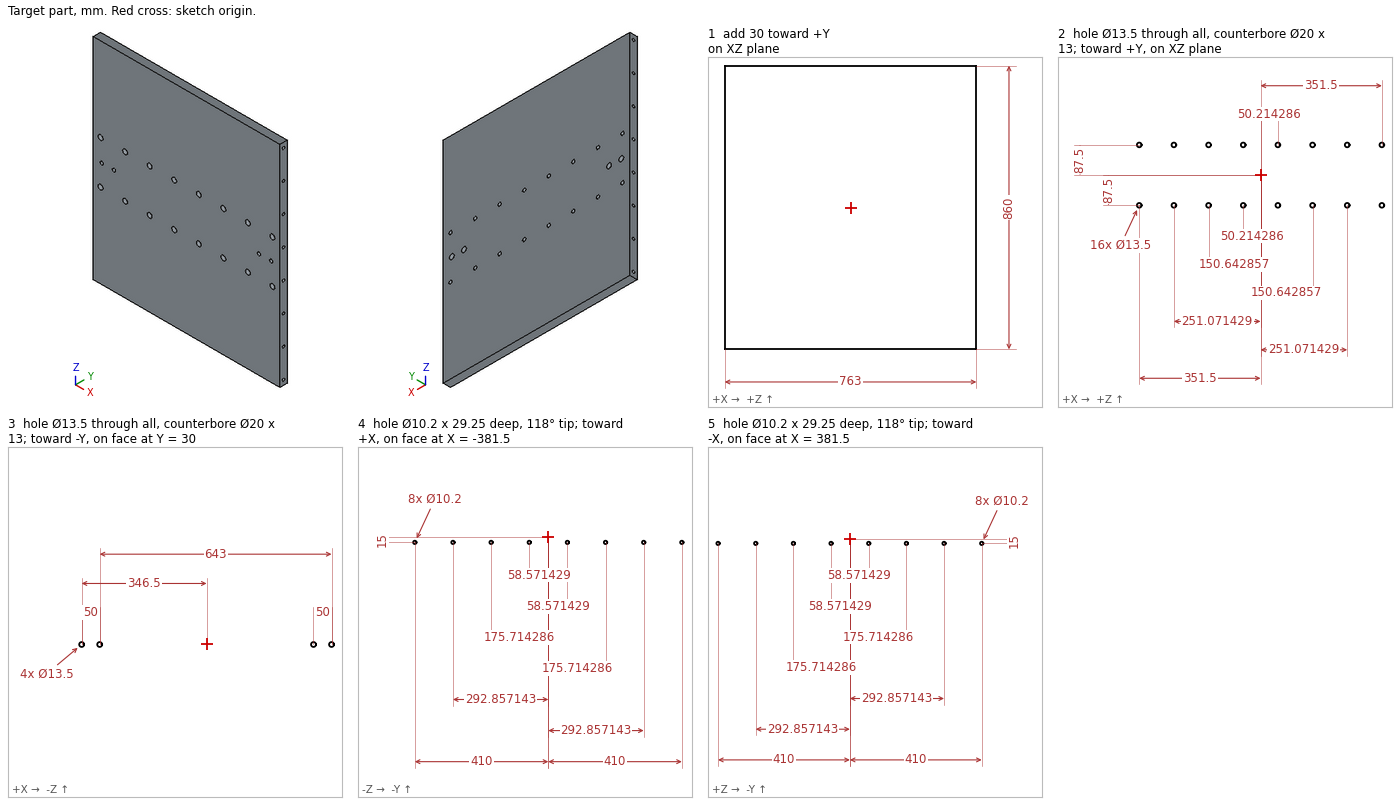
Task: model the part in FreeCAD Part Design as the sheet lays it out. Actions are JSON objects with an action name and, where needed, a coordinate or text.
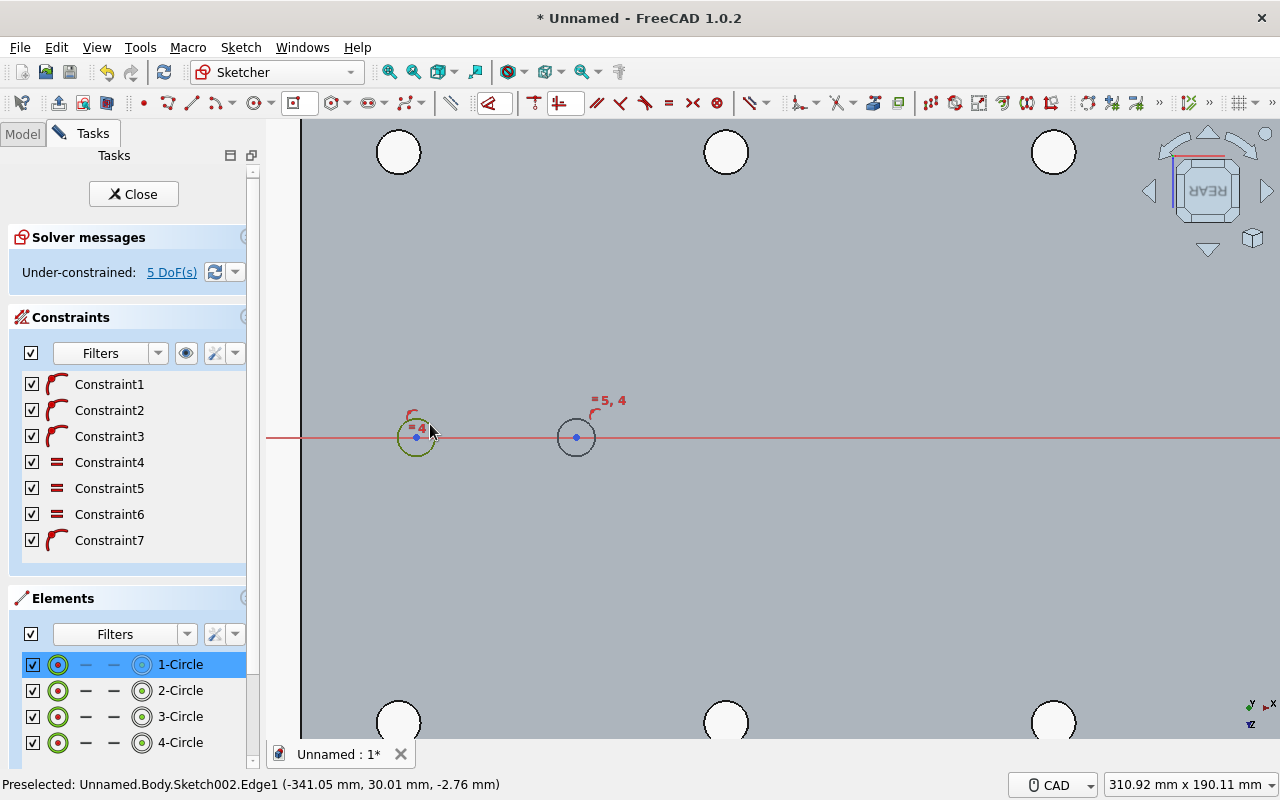
{"action": "key", "text": "k o"}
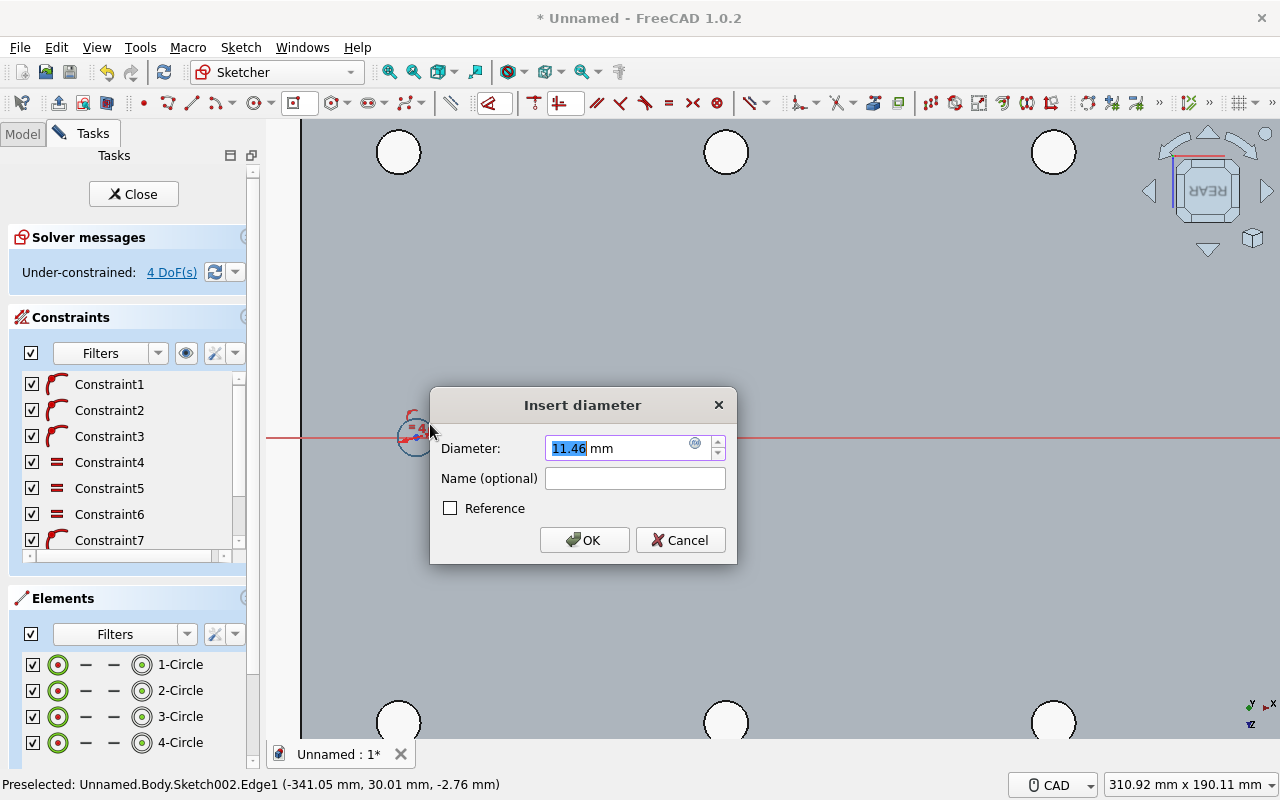
{"action": "type", "text": "13.5"}
{"action": "key", "text": "Return"}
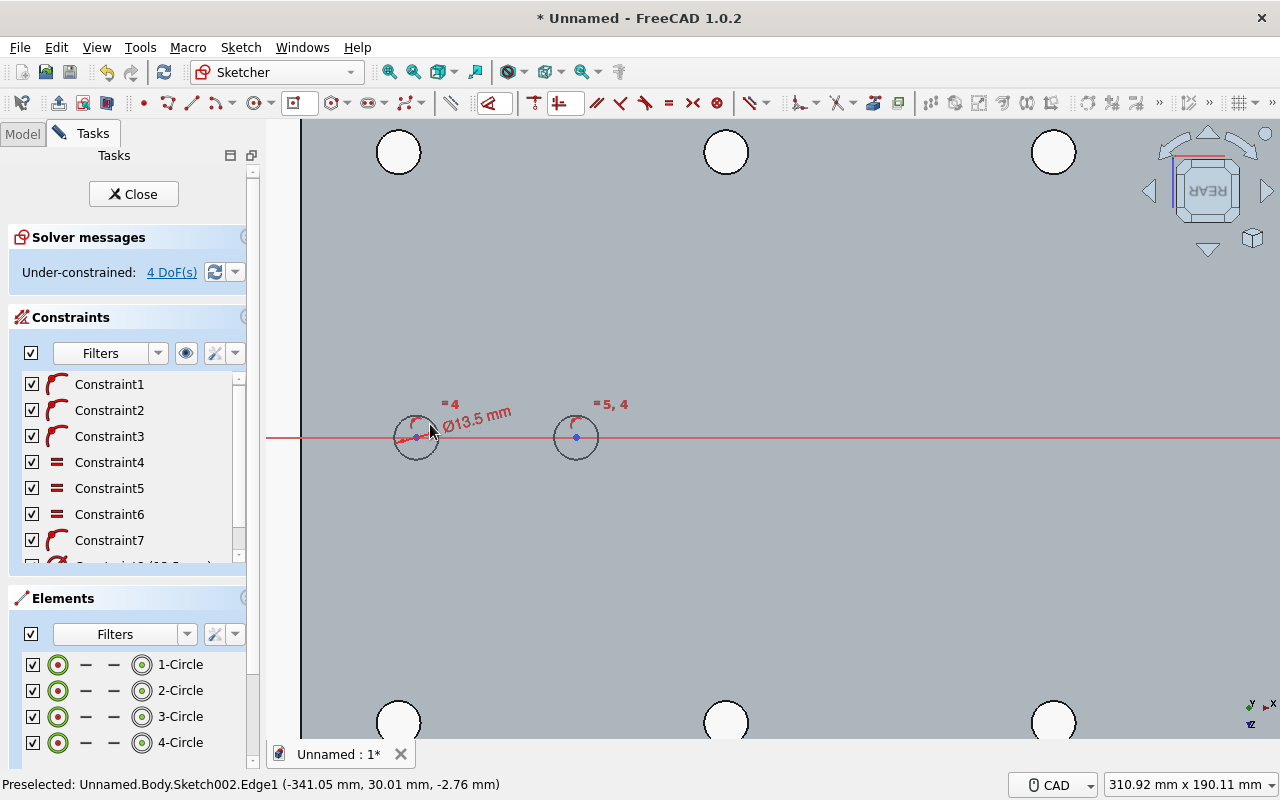
{"action": "scroll", "coordinate": [429, 426], "scroll_direction": "down", "scroll_amount": 7}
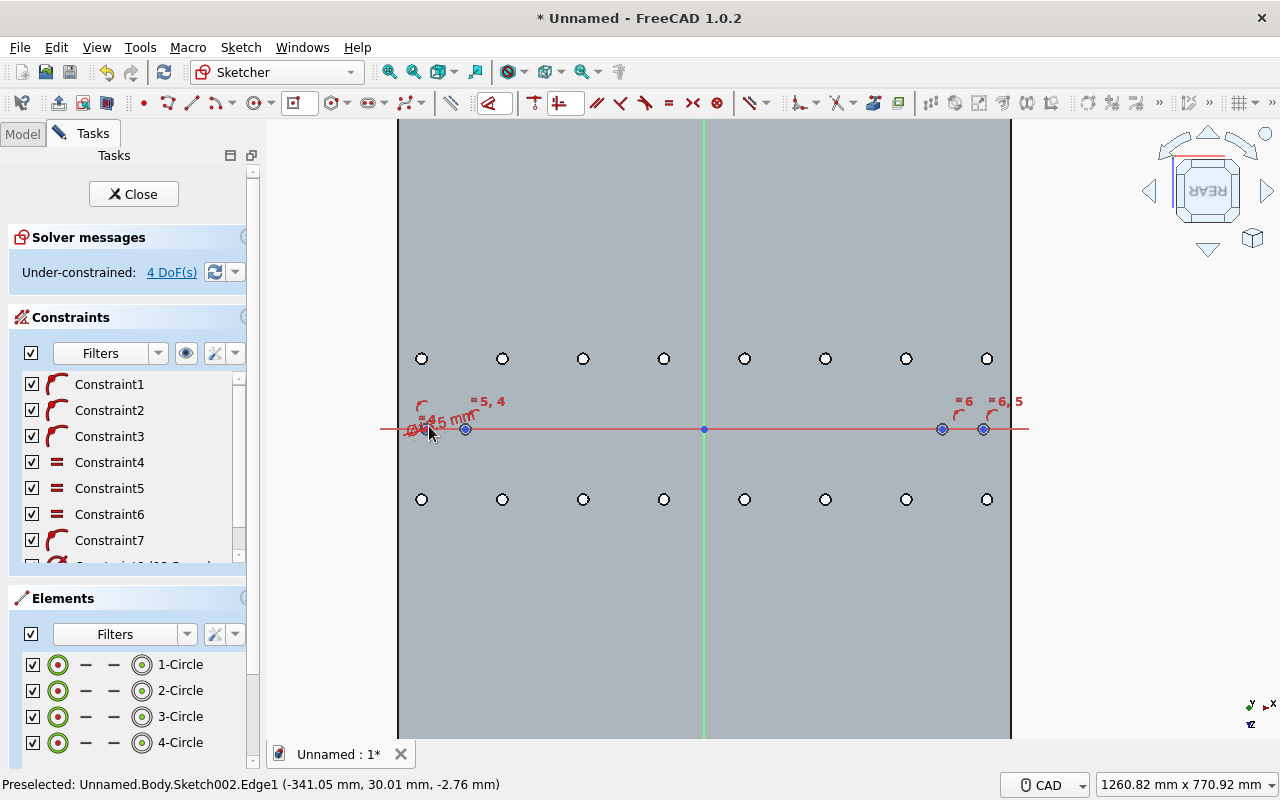
{"action": "left_click", "coordinate": [426, 429]}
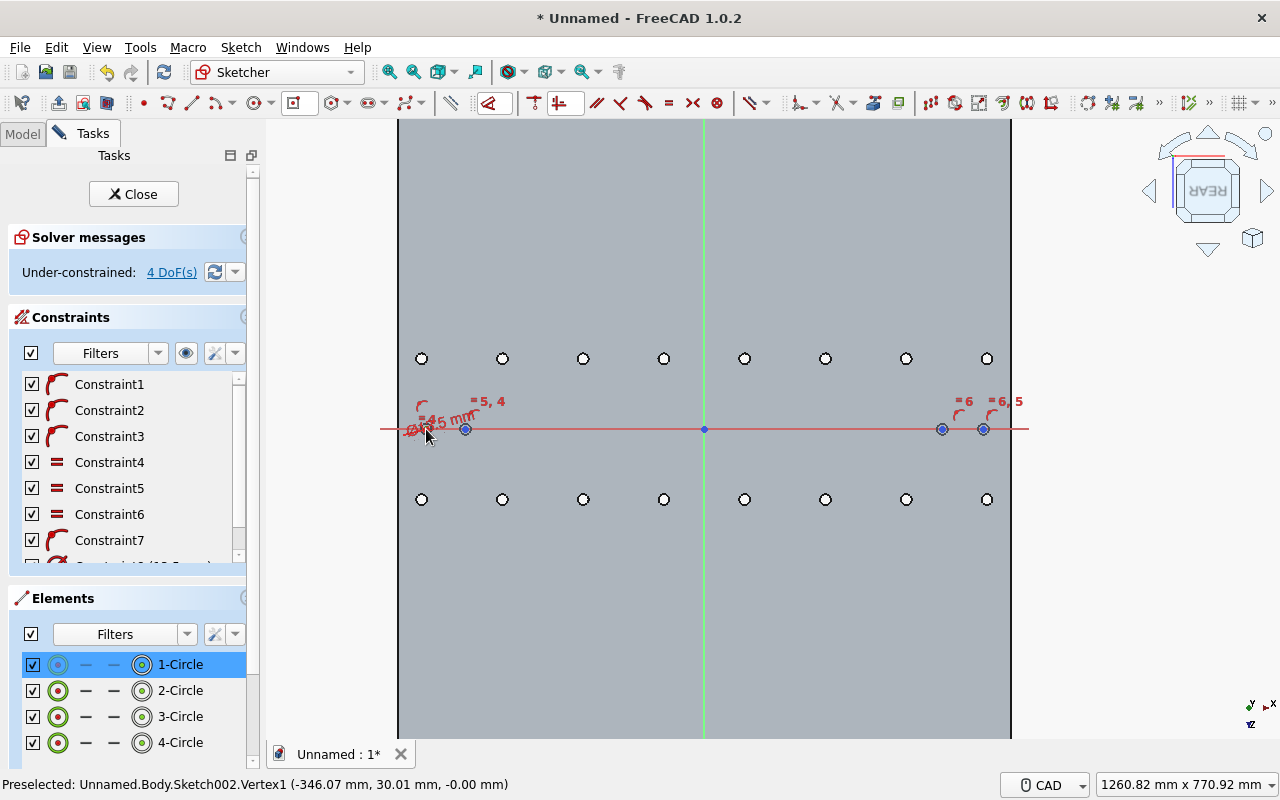
{"action": "left_click", "coordinate": [465, 429]}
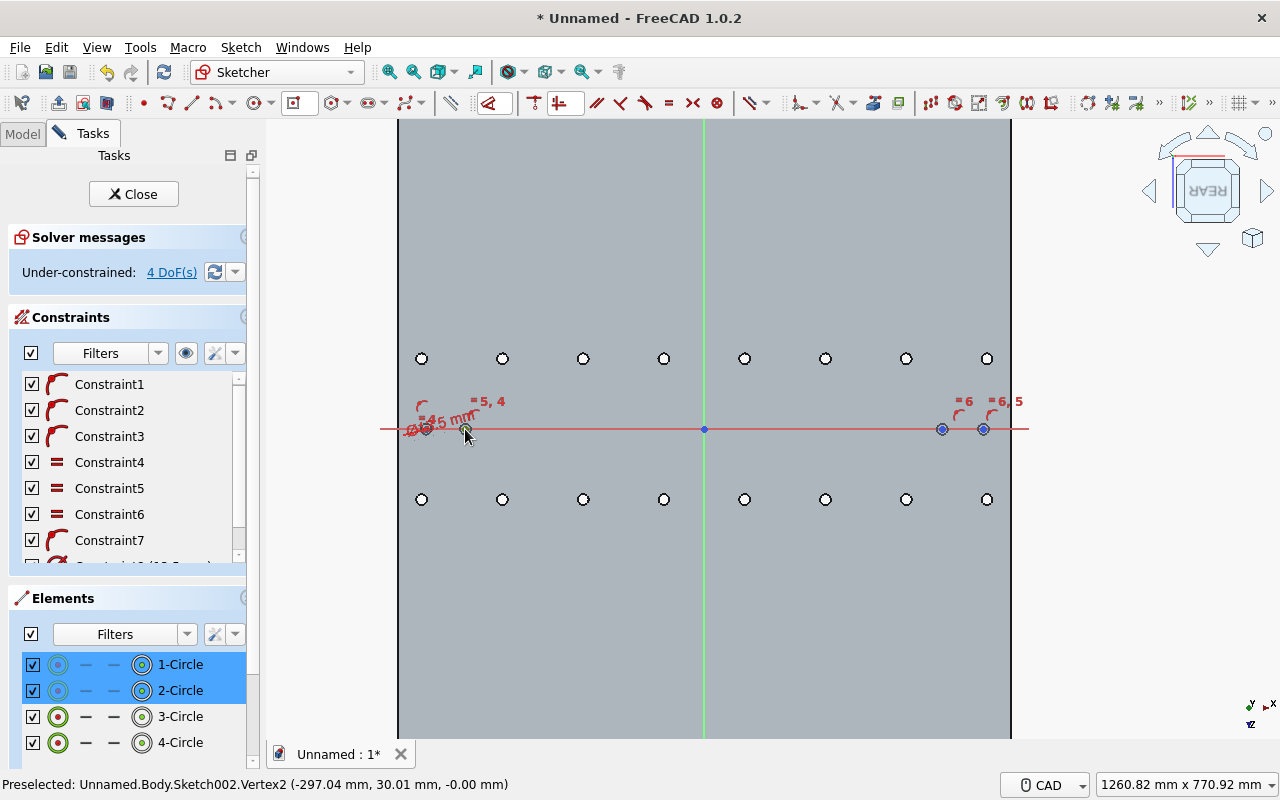
{"action": "left_click", "coordinate": [506, 104]}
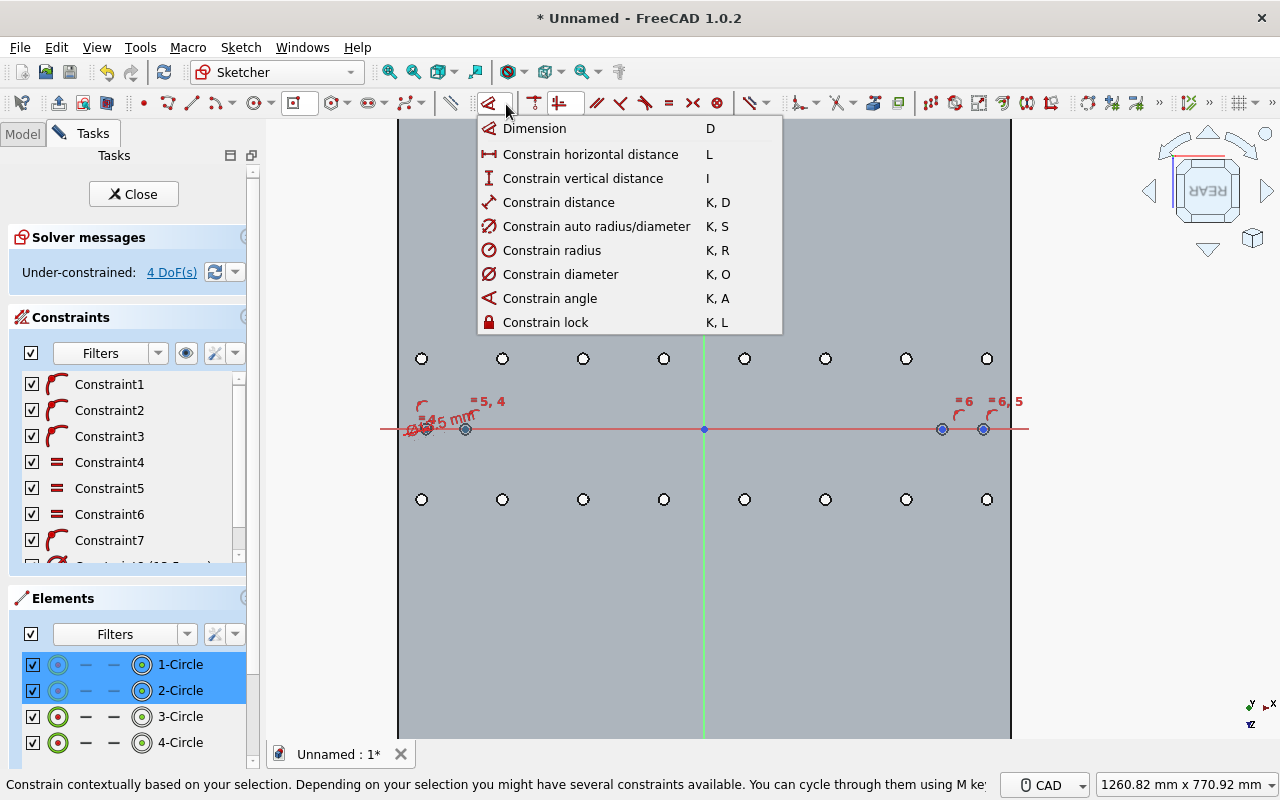
{"action": "left_click", "coordinate": [630, 154]}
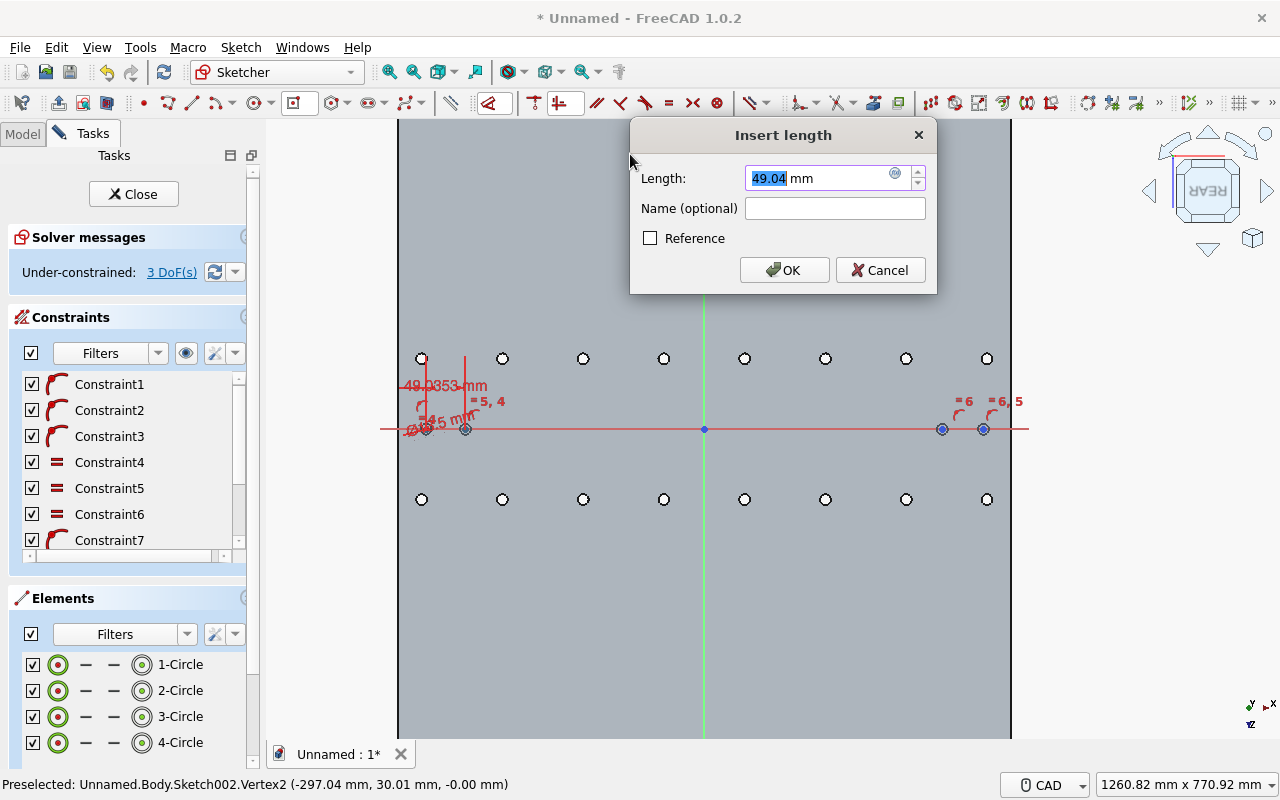
{"action": "type", "text": "50"}
{"action": "key", "text": "Return"}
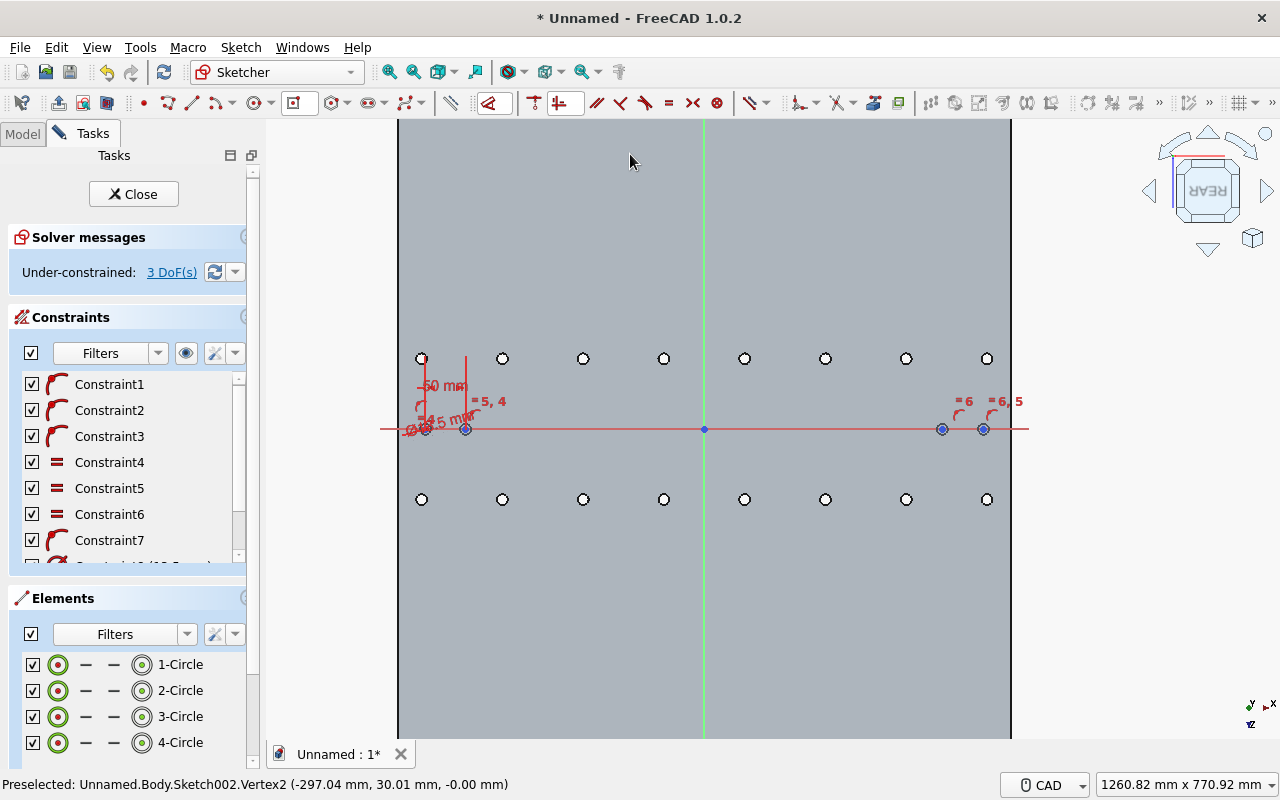
{"action": "left_click", "coordinate": [983, 429]}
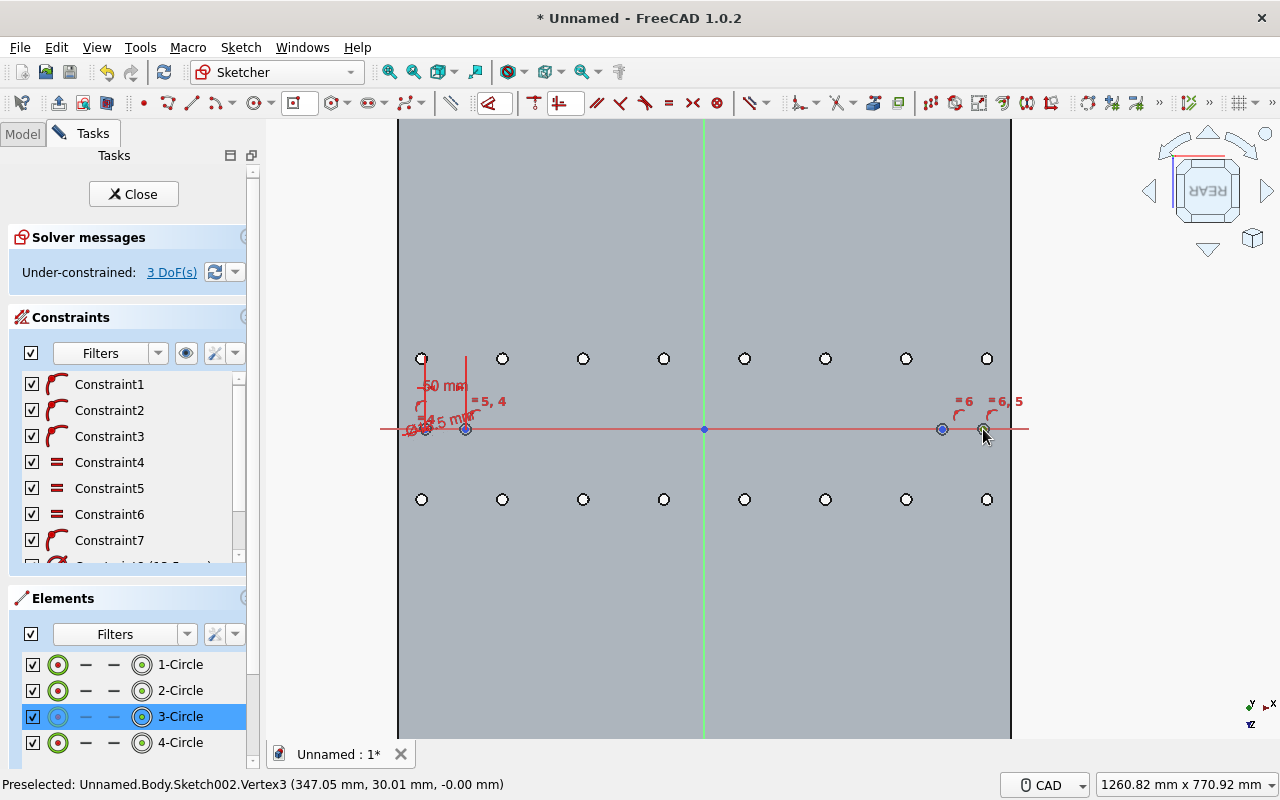
{"action": "left_click", "coordinate": [942, 429]}